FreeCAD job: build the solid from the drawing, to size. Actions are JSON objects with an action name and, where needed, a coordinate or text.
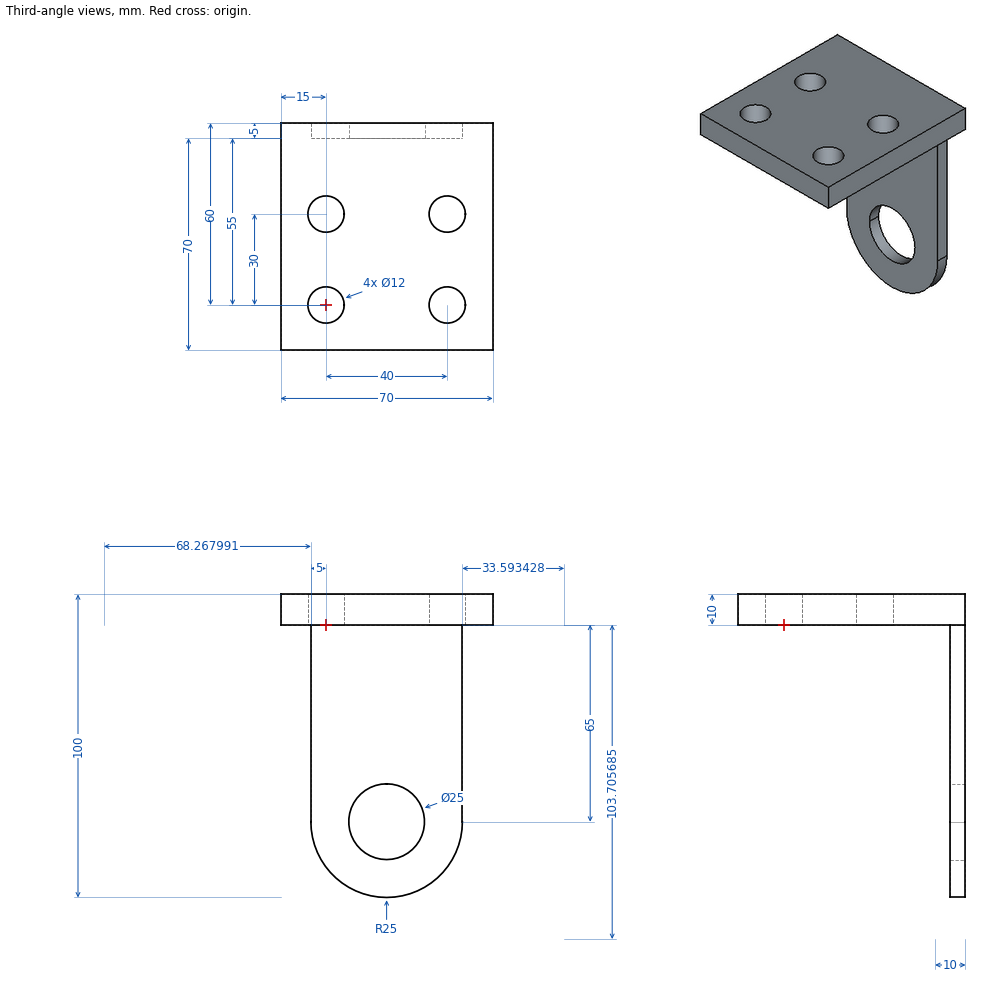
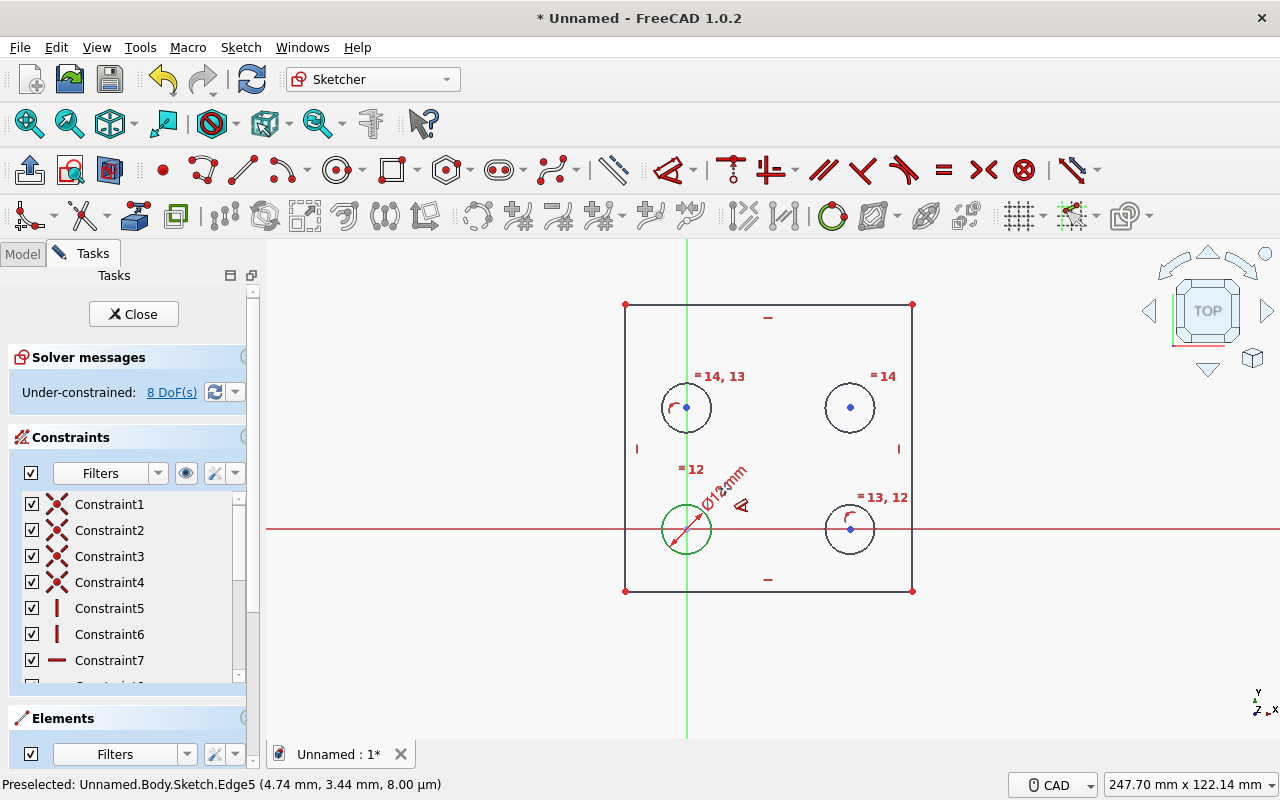
{"action": "left_click", "coordinate": [625, 391]}
{"action": "left_click", "coordinate": [591, 449]}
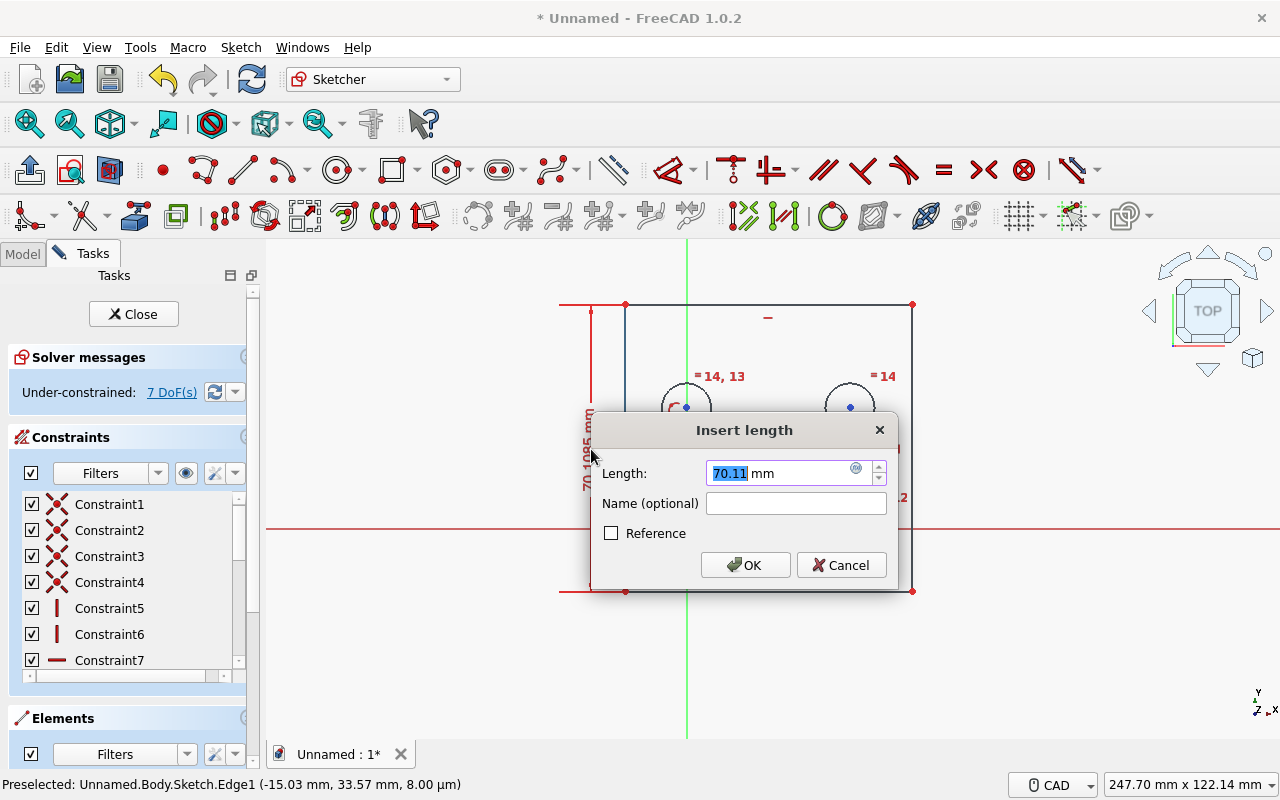
{"action": "type", "text": "70"}
{"action": "key", "text": "Return"}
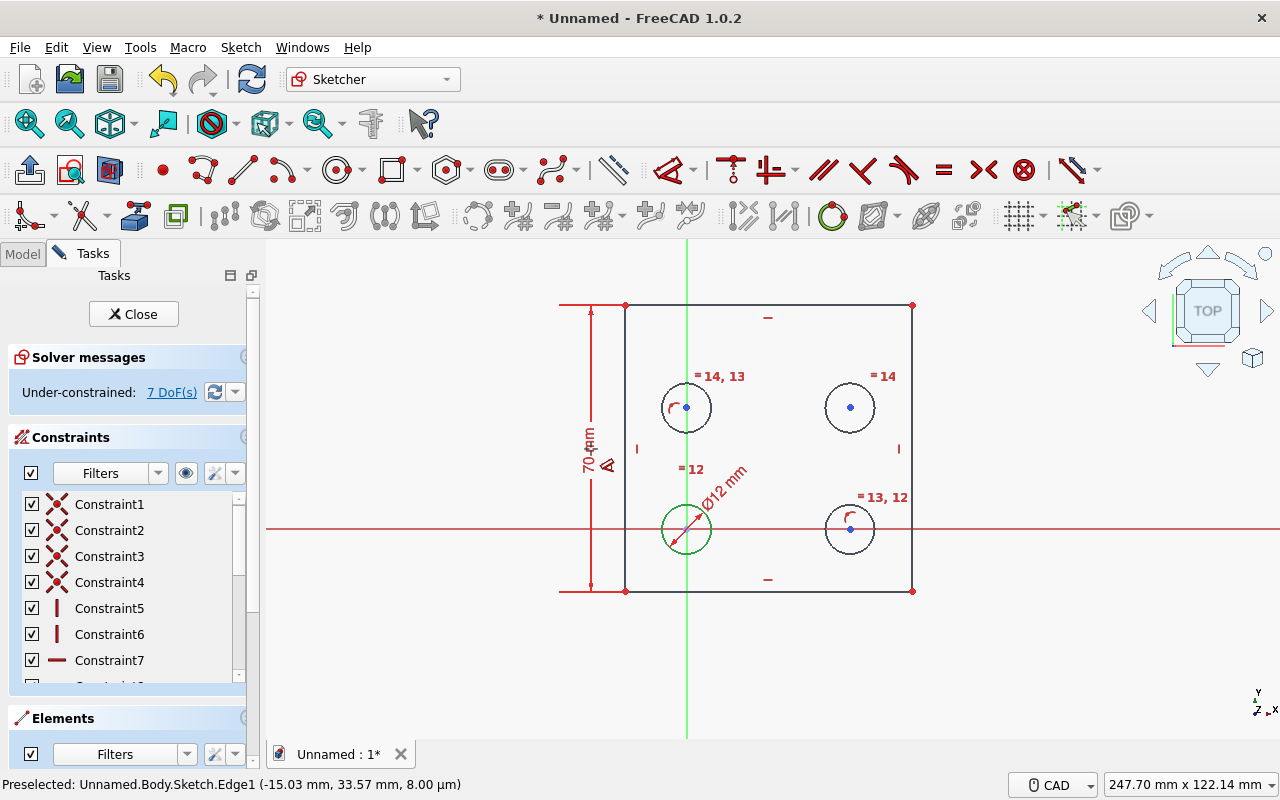
{"action": "left_click", "coordinate": [711, 592]}
{"action": "left_click", "coordinate": [768, 626]}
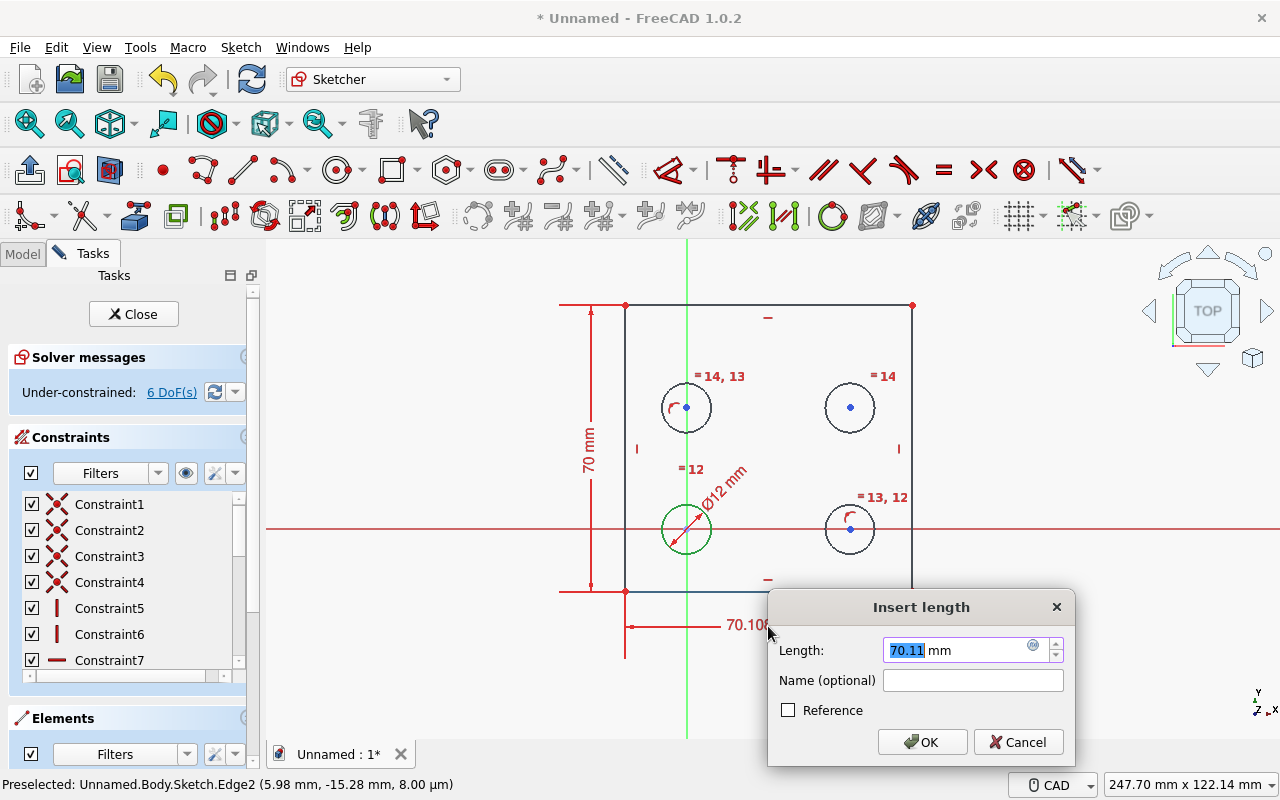
{"action": "type", "text": "70"}
{"action": "key", "text": "Return"}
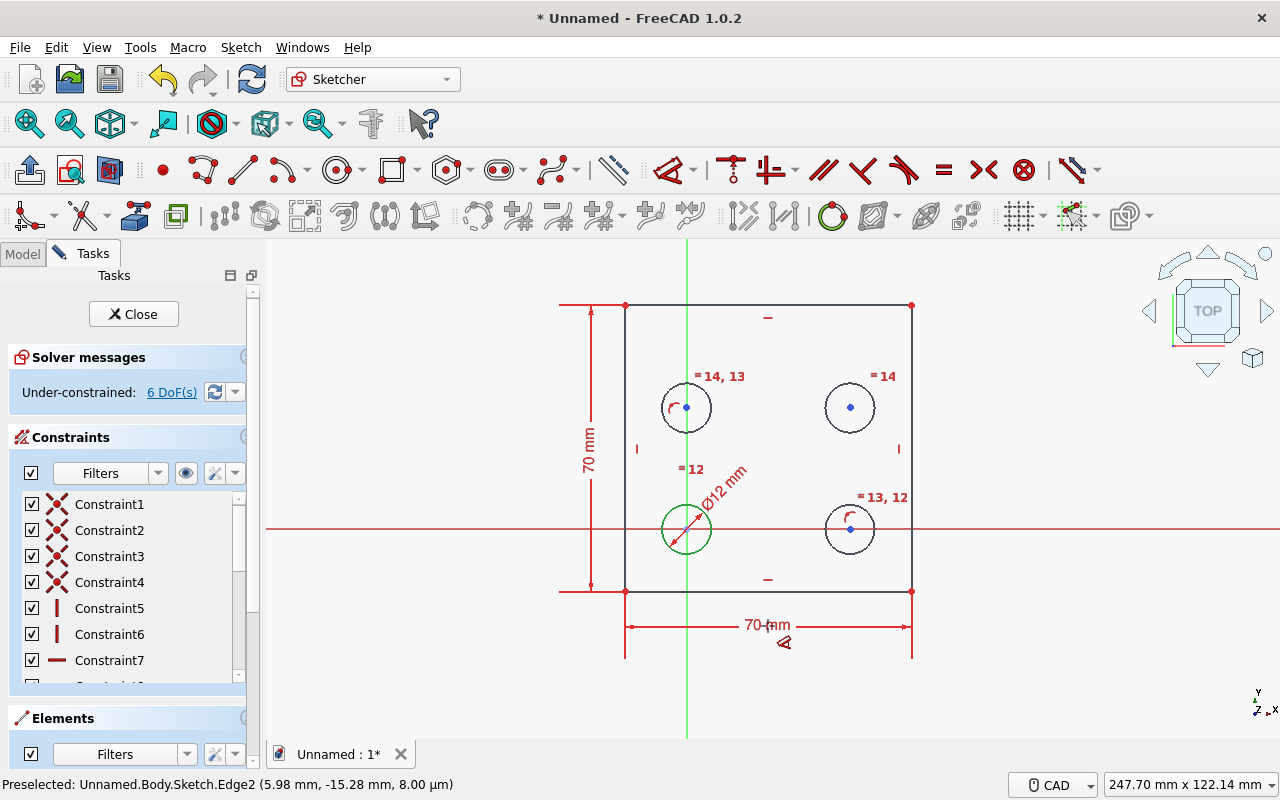
{"action": "left_click", "coordinate": [850, 529]}
{"action": "left_click", "coordinate": [768, 563]}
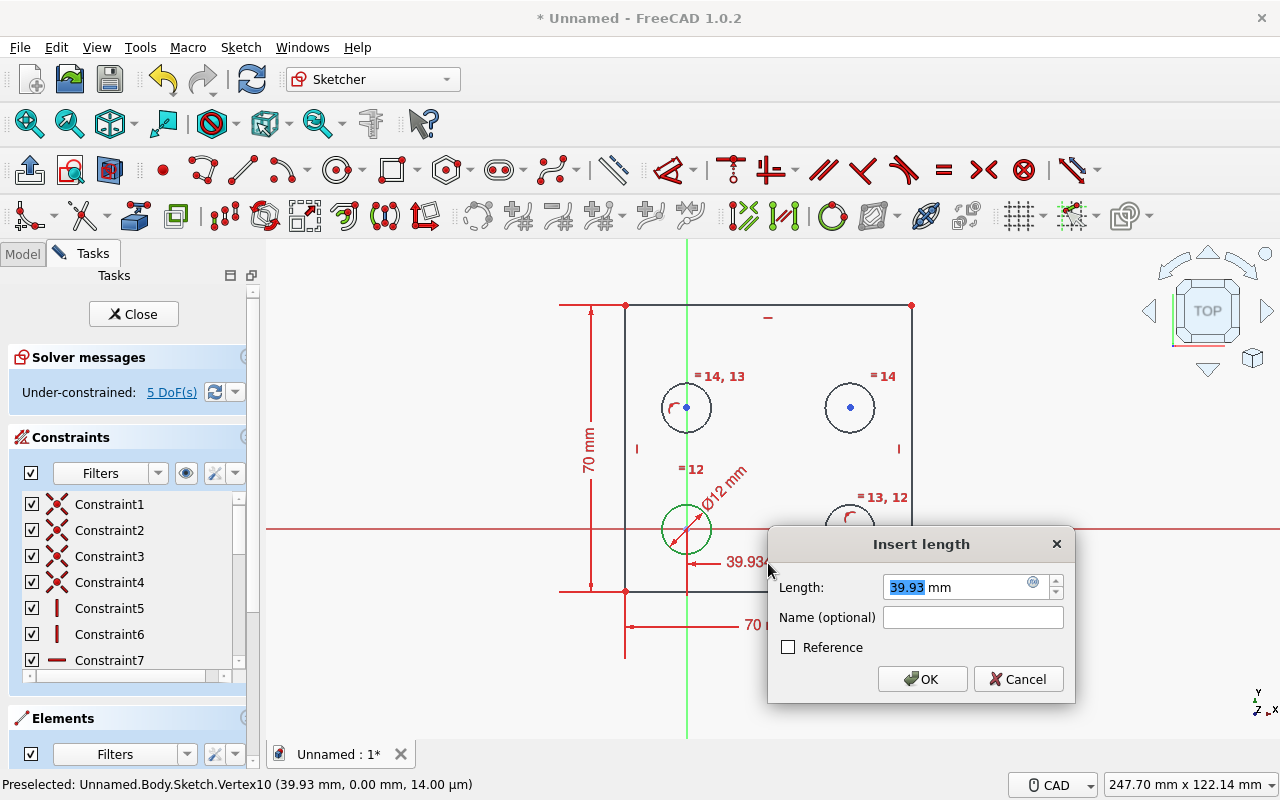
{"action": "type", "text": "40"}
{"action": "key", "text": "Return"}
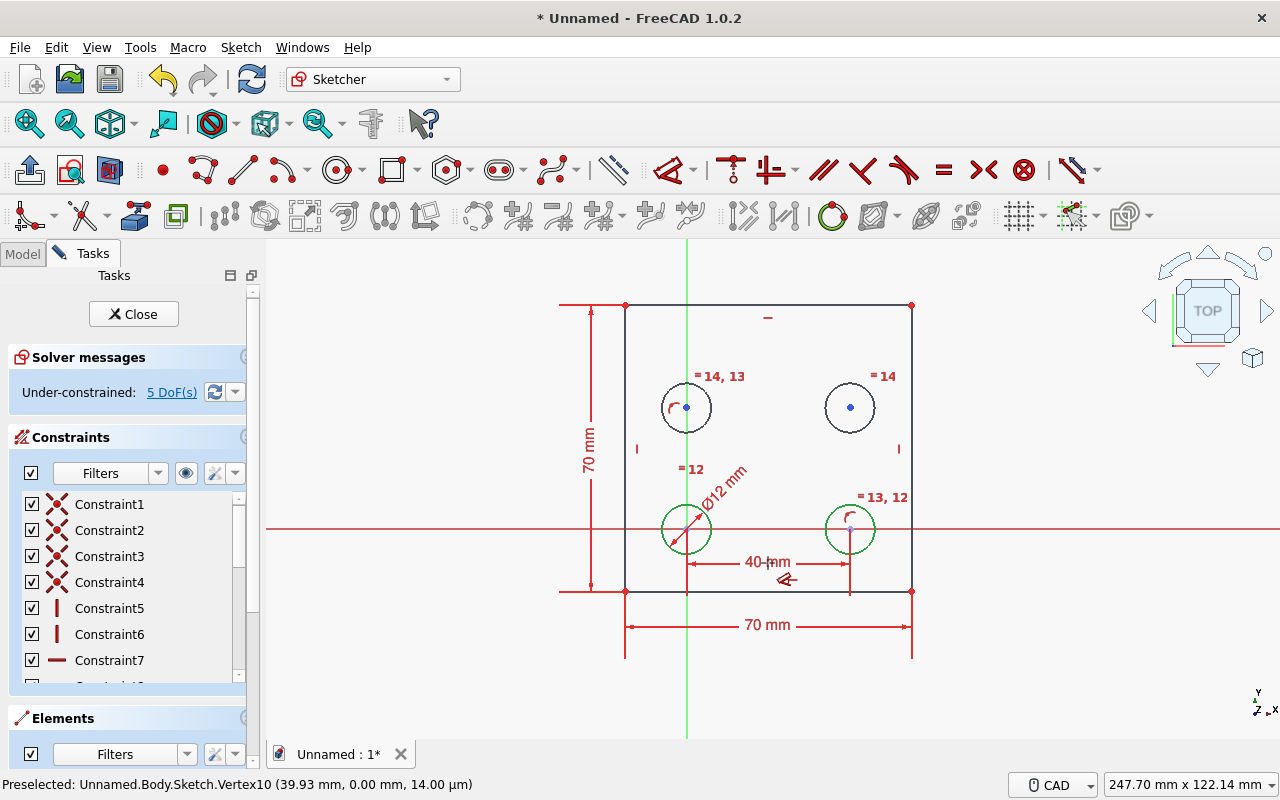
{"action": "left_click", "coordinate": [687, 408]}
{"action": "left_click", "coordinate": [653, 469]}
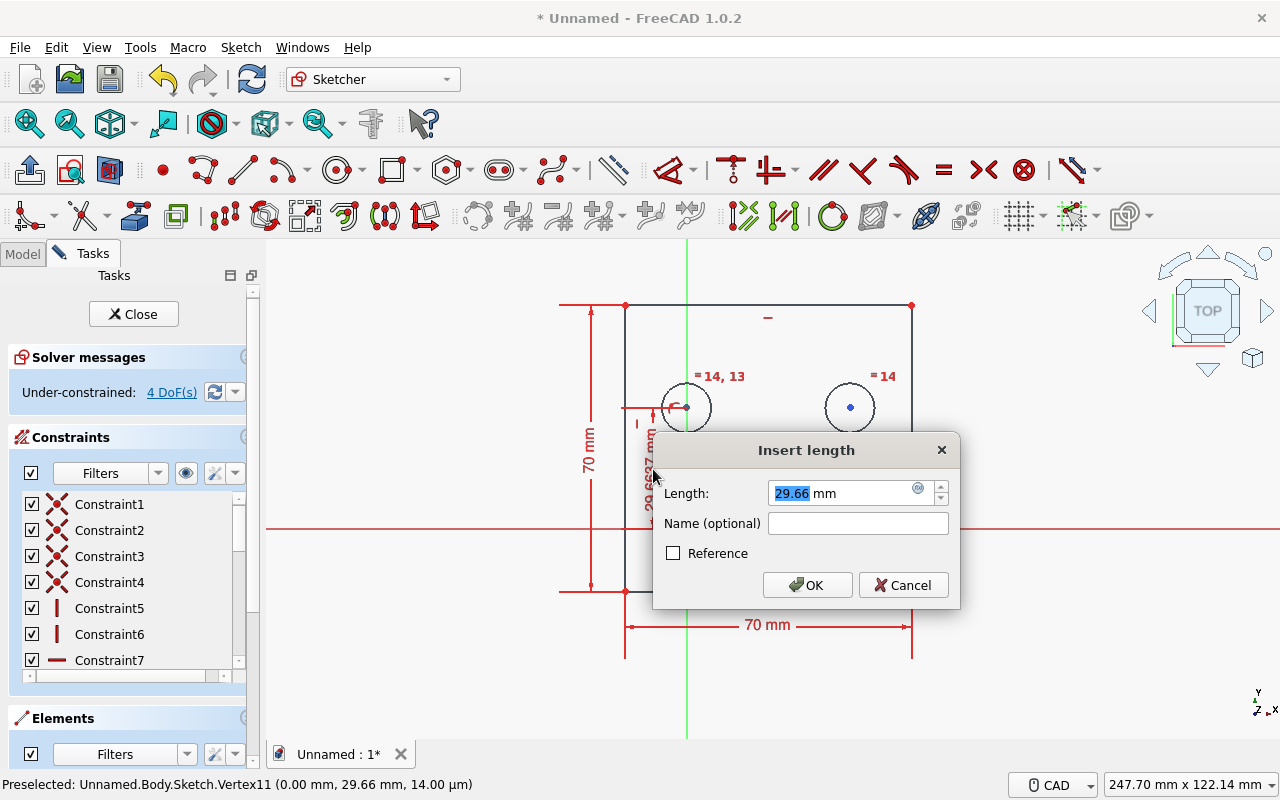
{"action": "type", "text": "30"}
{"action": "key", "text": "Return"}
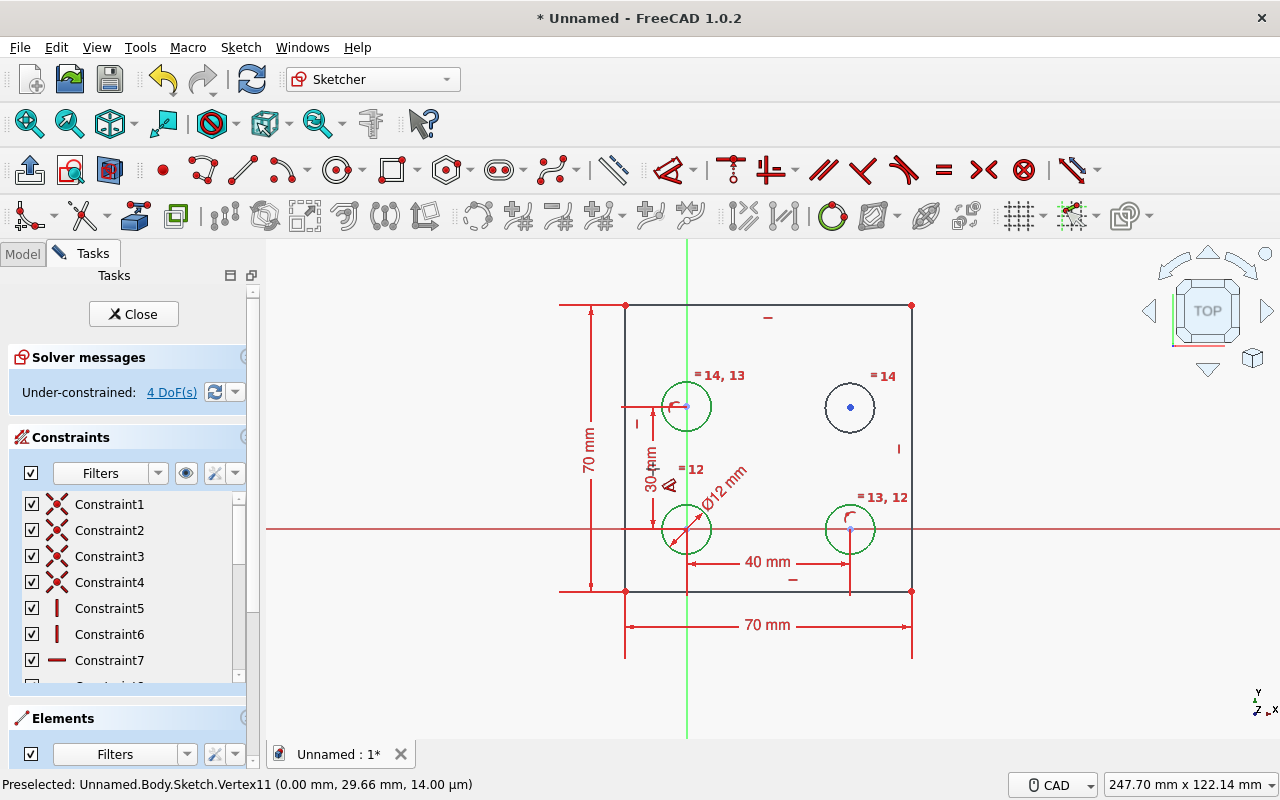
{"action": "left_click", "coordinate": [850, 408]}
{"action": "left_click", "coordinate": [768, 374]}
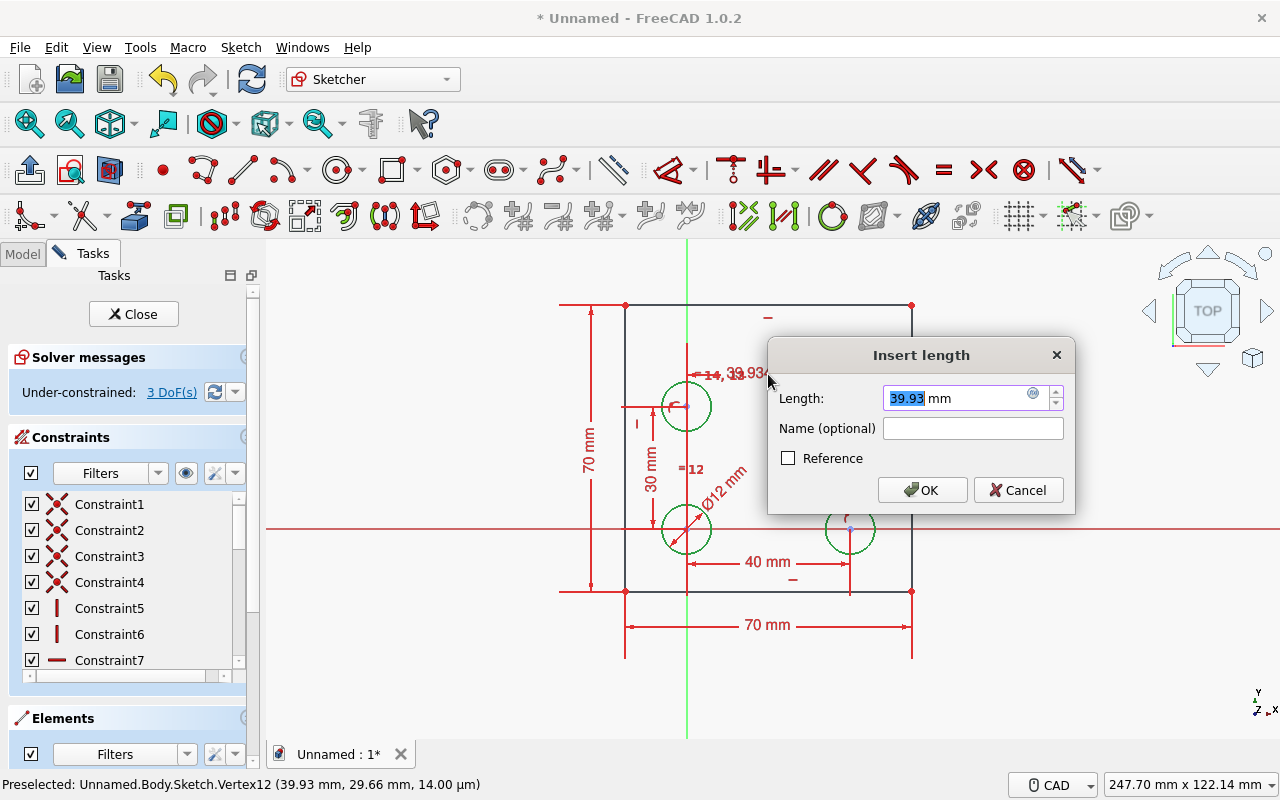
{"action": "type", "text": "40"}
{"action": "key", "text": "Return"}